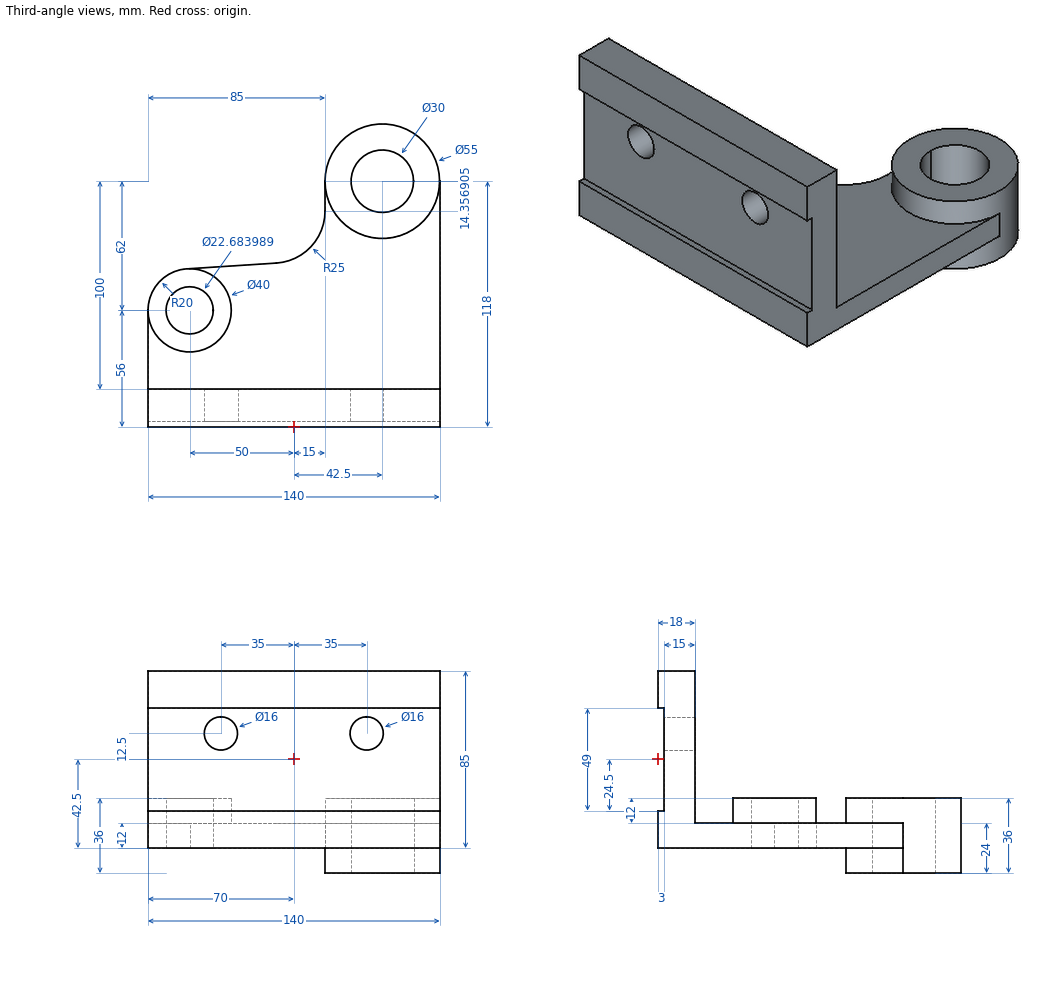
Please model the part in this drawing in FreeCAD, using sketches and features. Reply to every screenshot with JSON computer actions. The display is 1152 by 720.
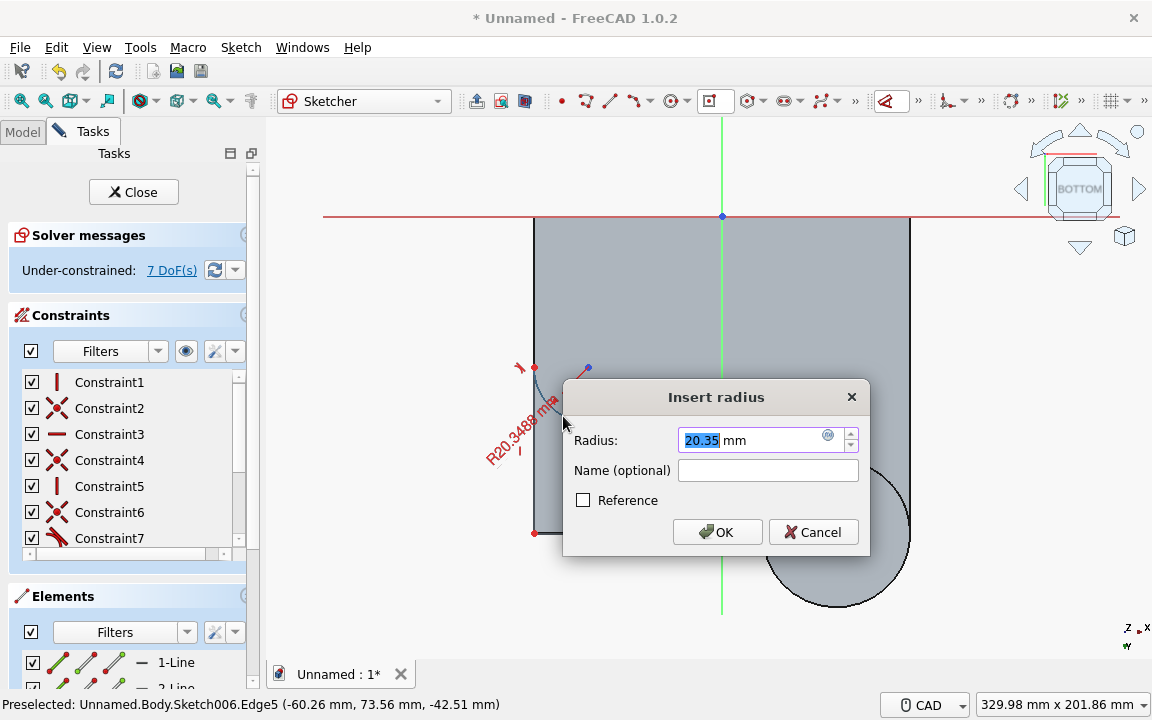
{"action": "type", "text": "20"}
{"action": "key", "text": "Return"}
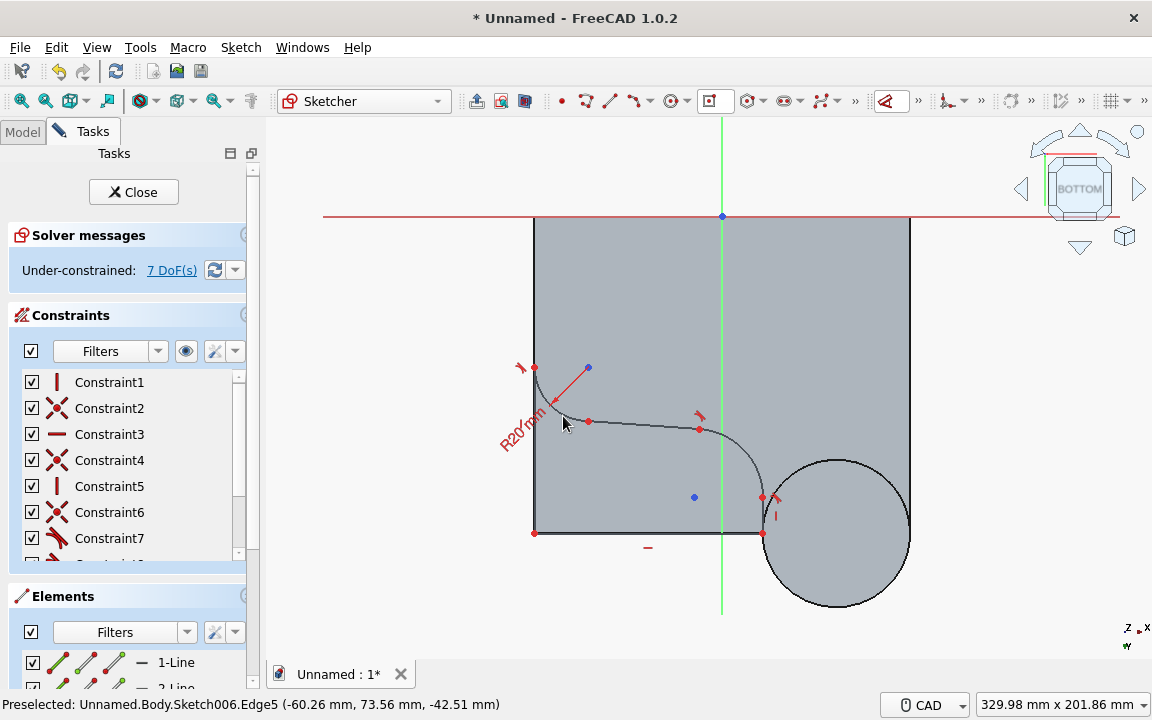
{"action": "left_click", "coordinate": [756, 468]}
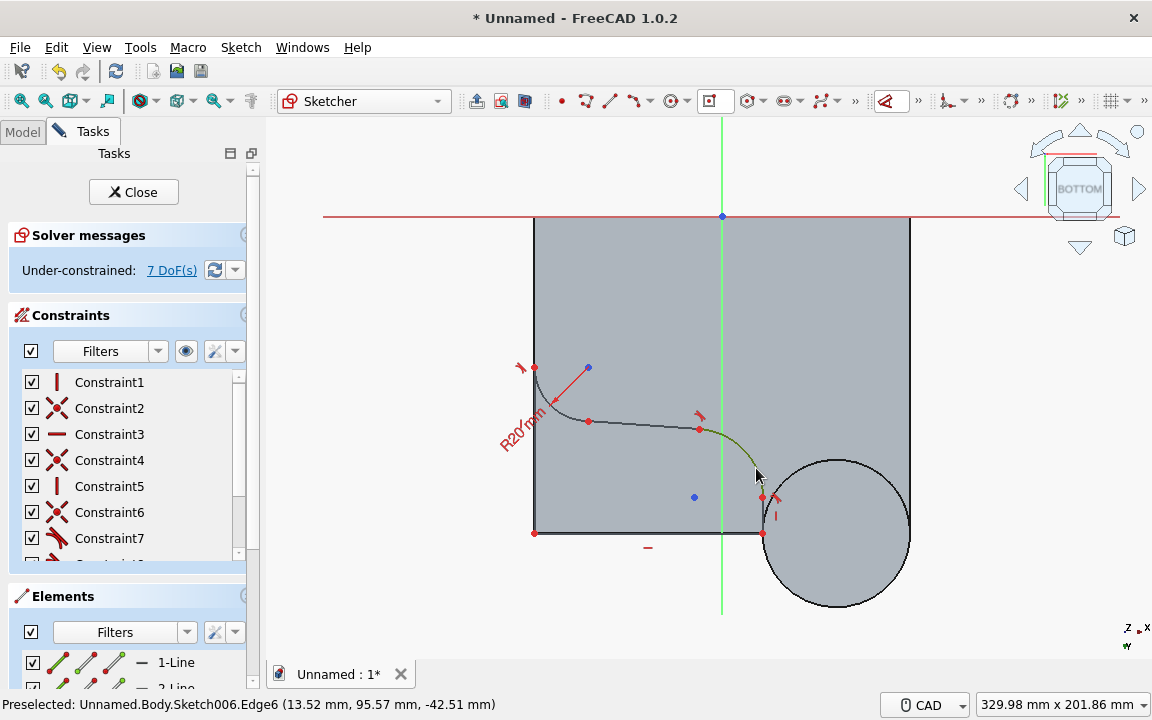
{"action": "key", "text": "k r"}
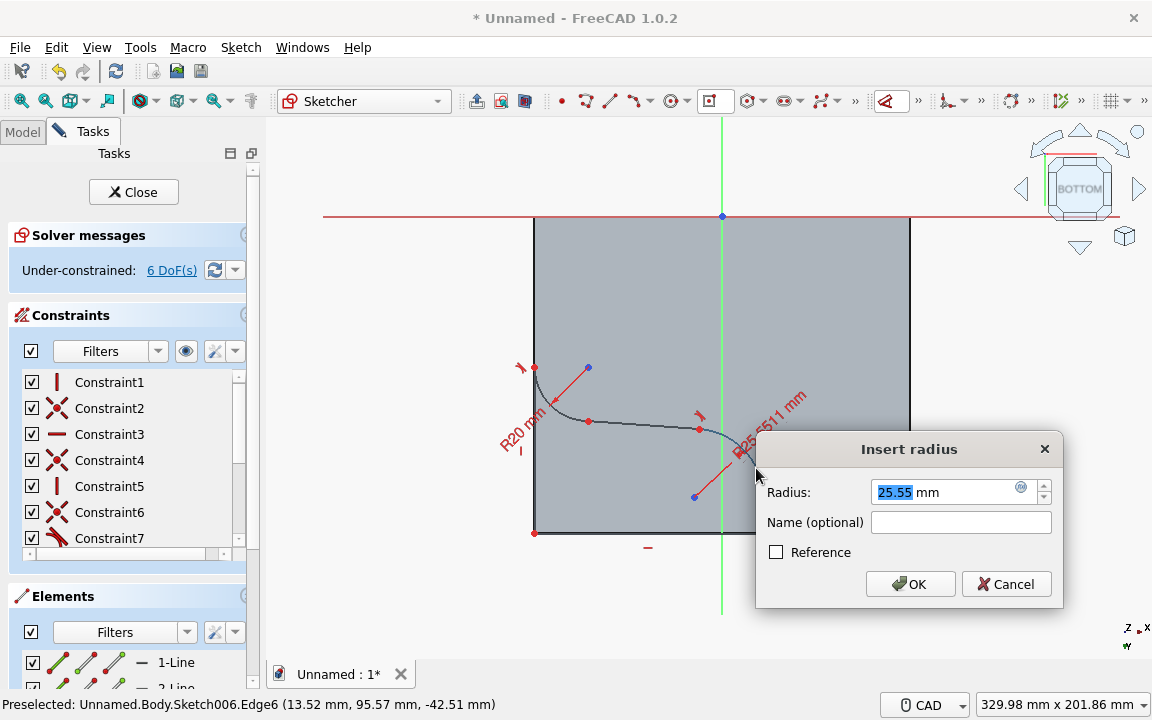
{"action": "type", "text": "25"}
{"action": "key", "text": "Return"}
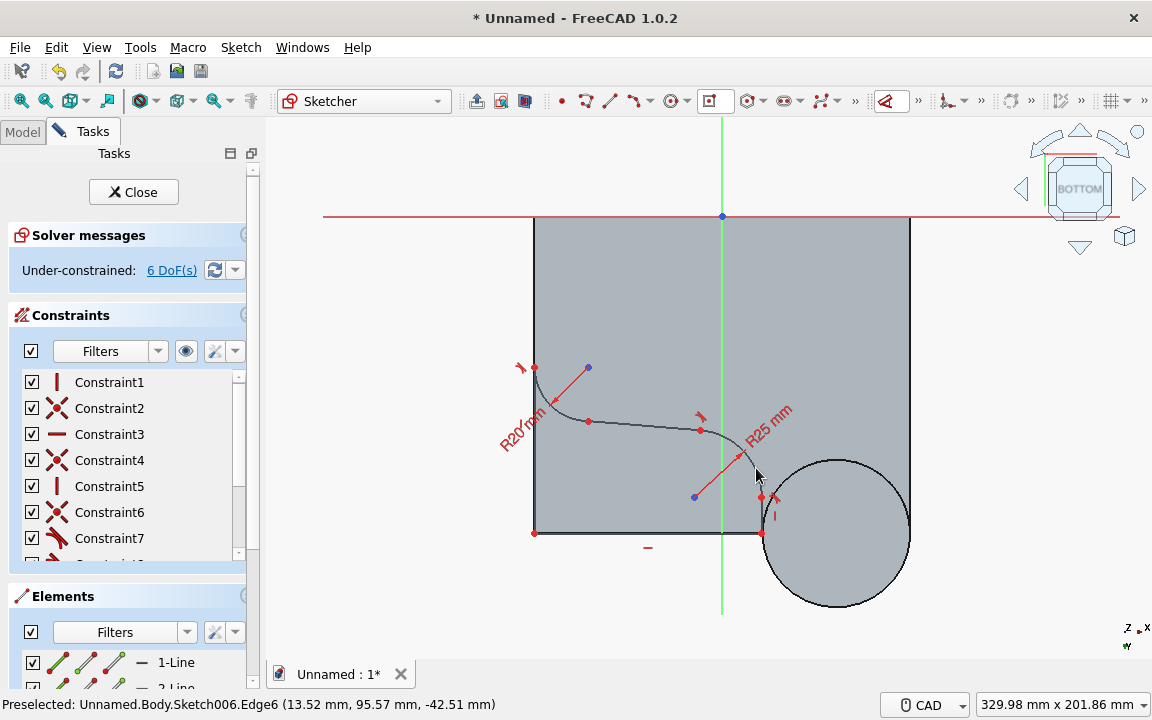
{"action": "left_click", "coordinate": [694, 534]}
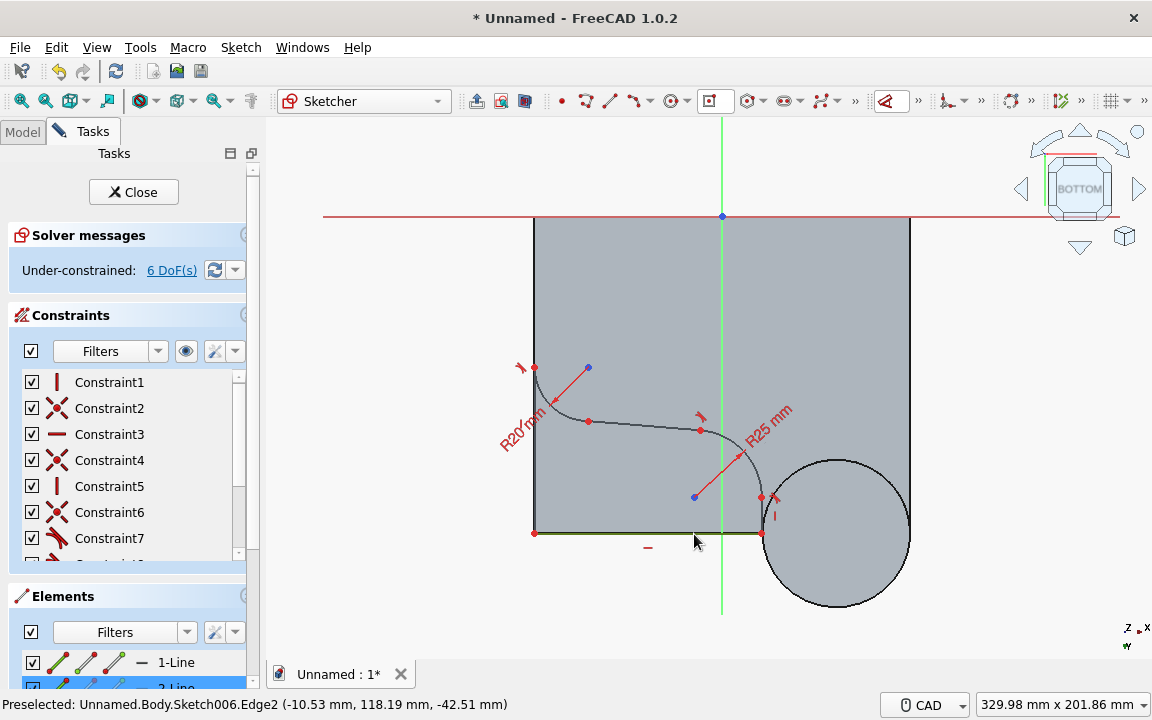
{"action": "key", "text": "l"}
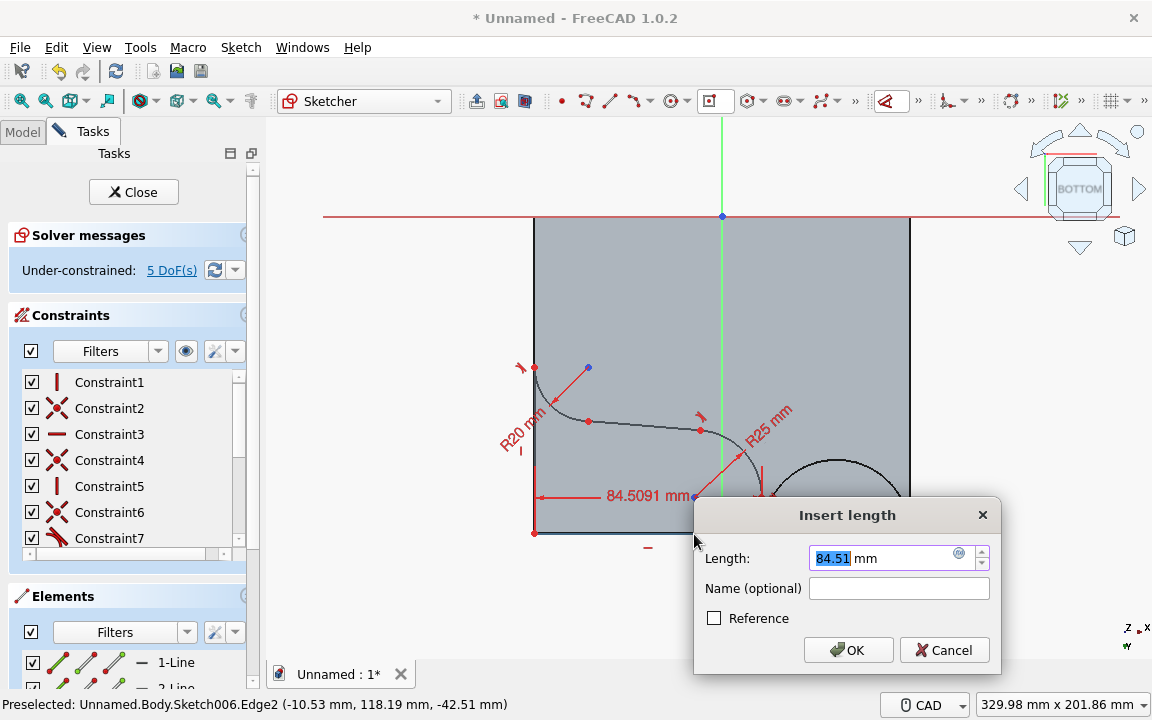
{"action": "type", "text": "85"}
{"action": "key", "text": "Return"}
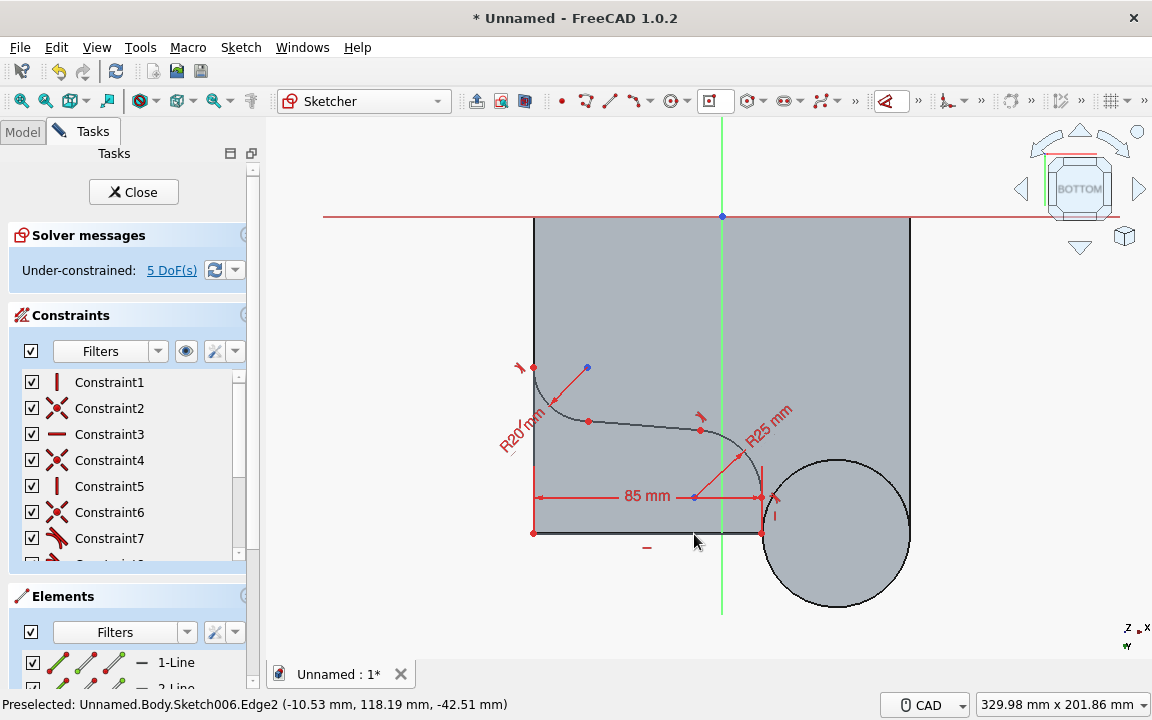
{"action": "left_click", "coordinate": [534, 484]}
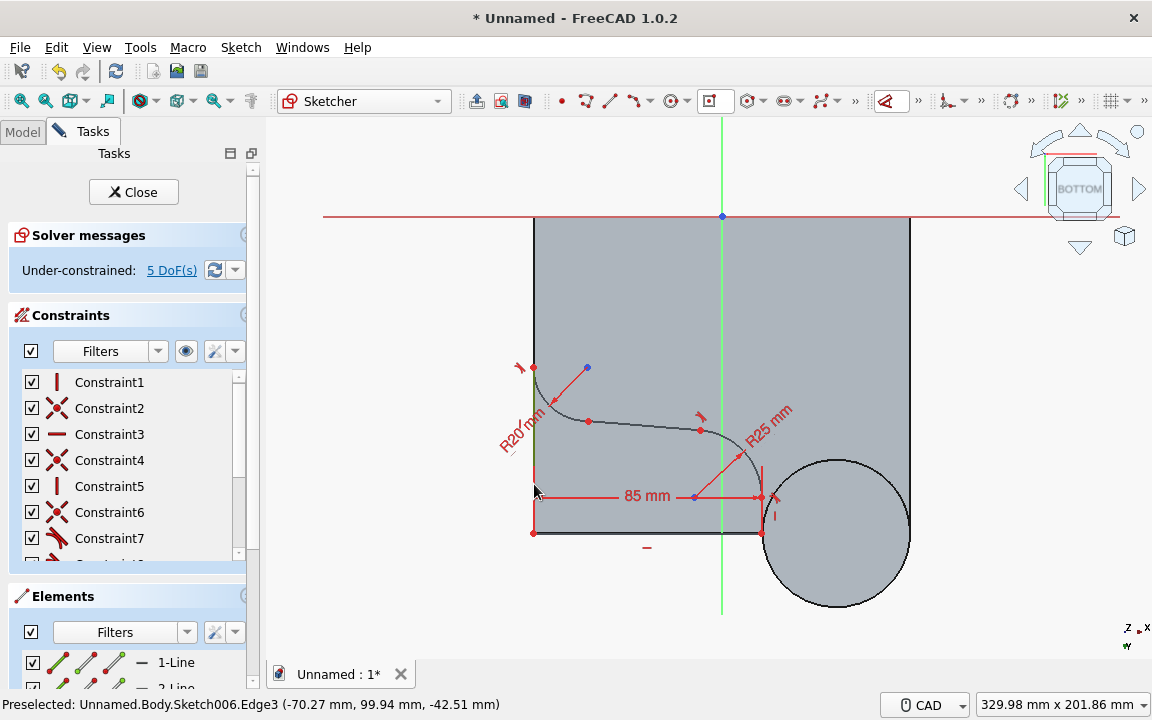
{"action": "left_click", "coordinate": [904, 102]}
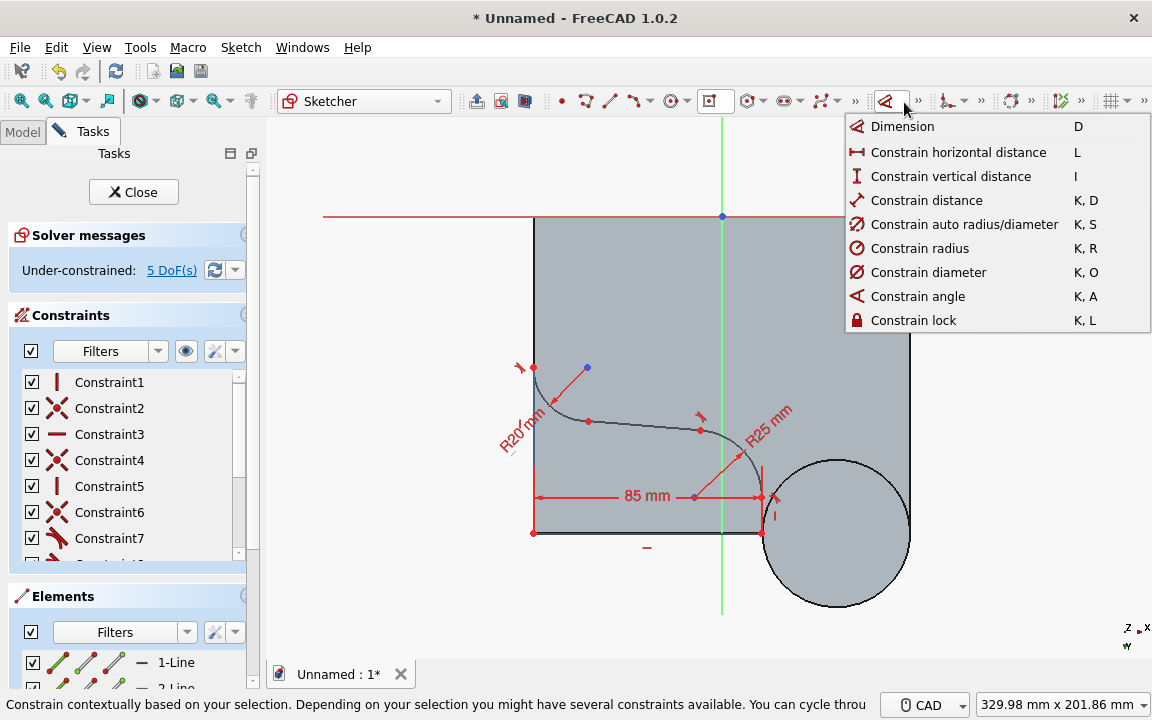
{"action": "left_click", "coordinate": [998, 176]}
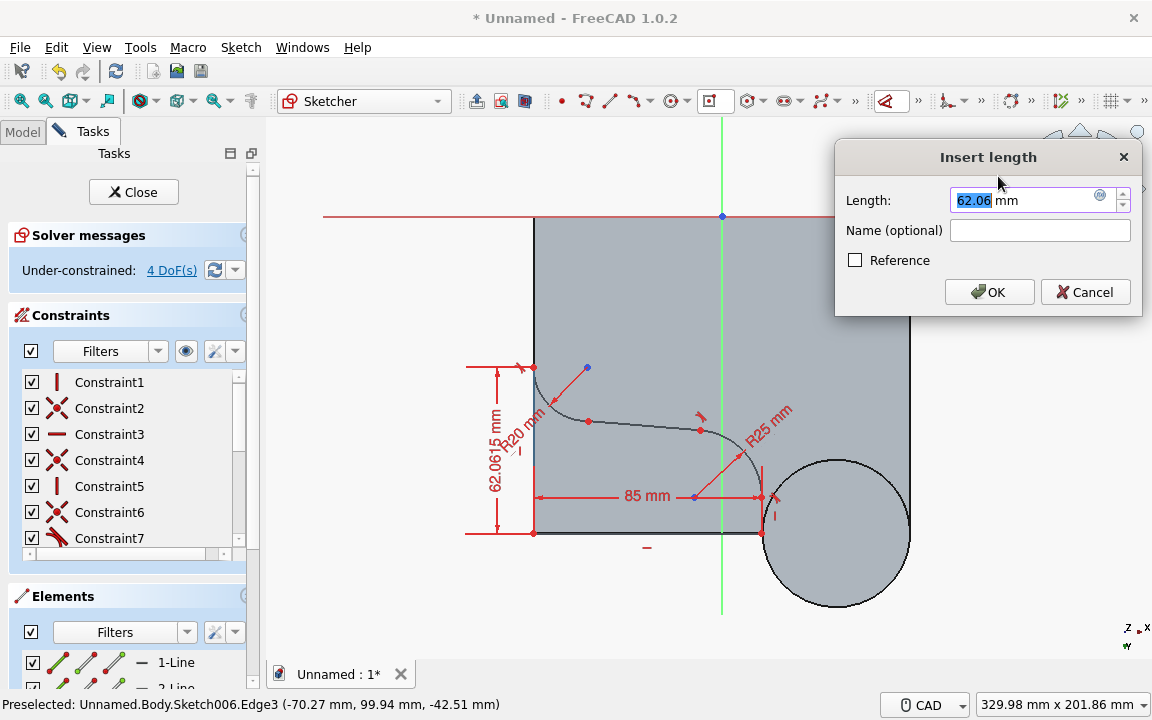
{"action": "type", "text": "62"}
{"action": "key", "text": "Return"}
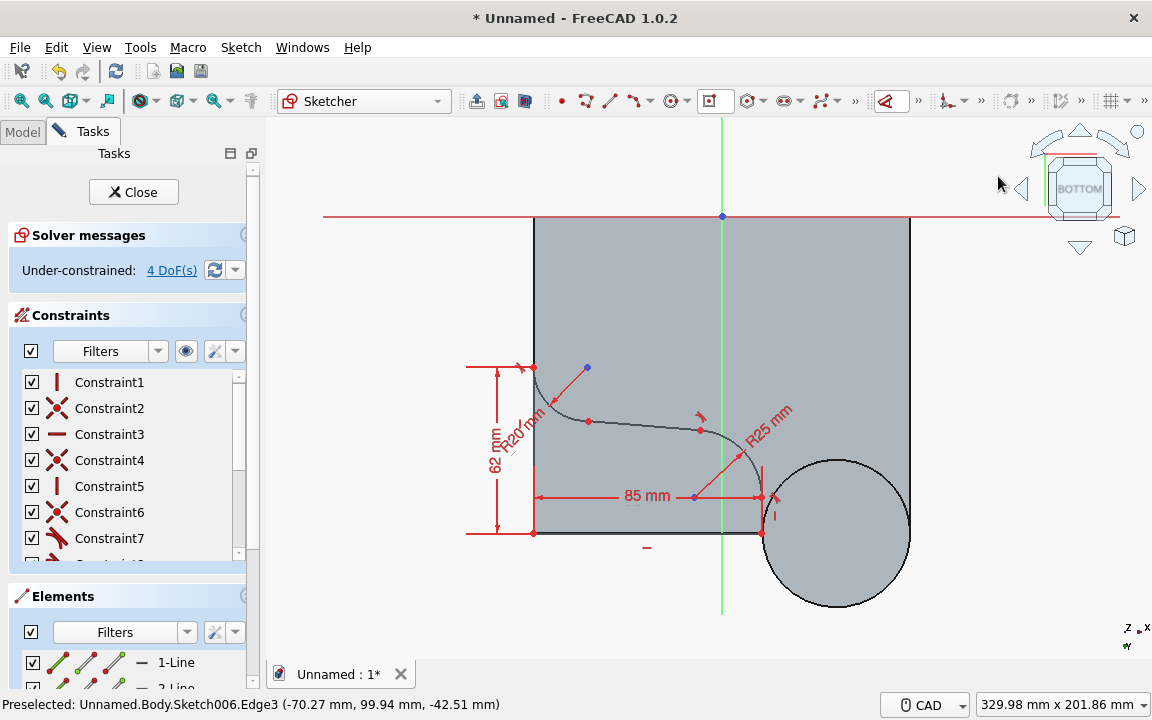
{"action": "left_click", "coordinate": [762, 497]}